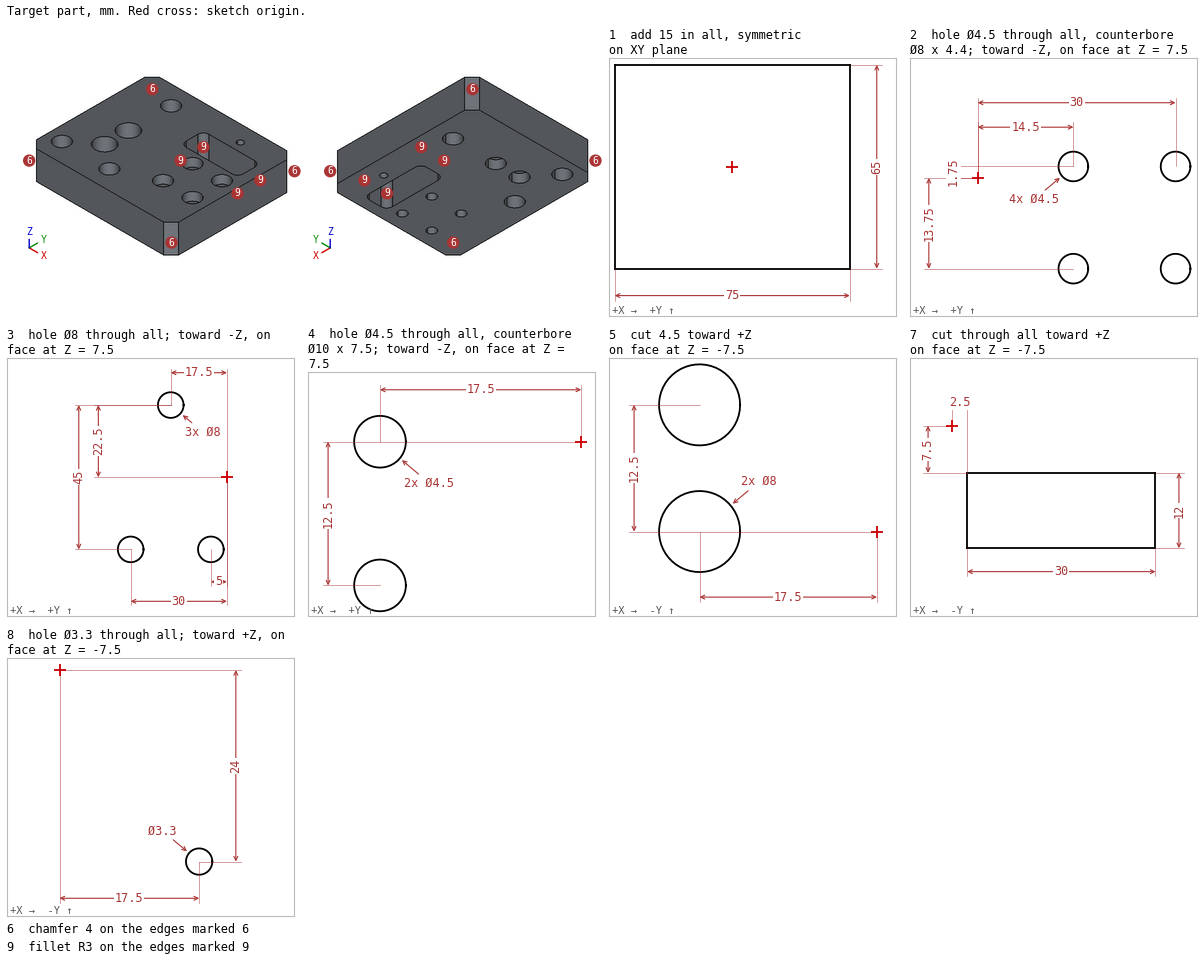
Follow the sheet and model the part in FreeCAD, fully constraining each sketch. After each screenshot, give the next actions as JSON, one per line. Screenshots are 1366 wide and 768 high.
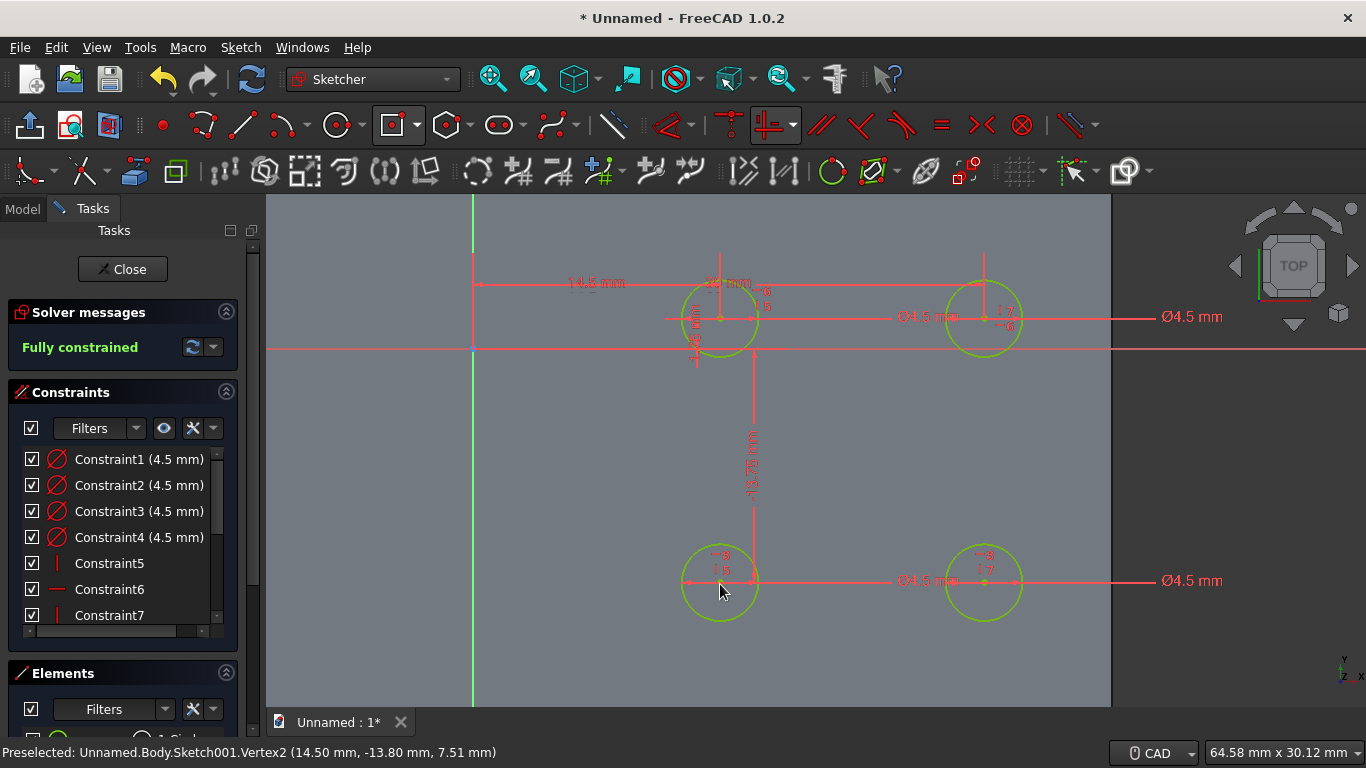
{"action": "left_click", "coordinate": [123, 269]}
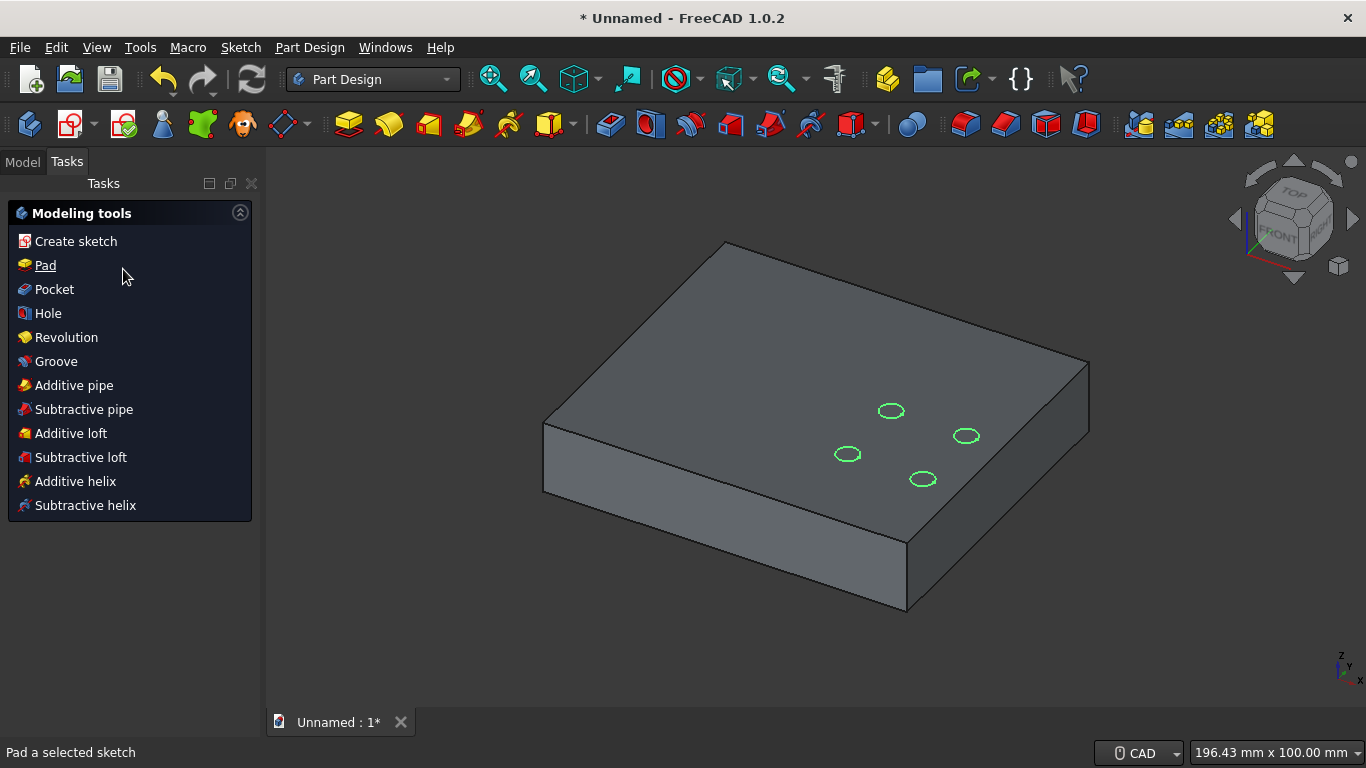
{"action": "left_click", "coordinate": [652, 124]}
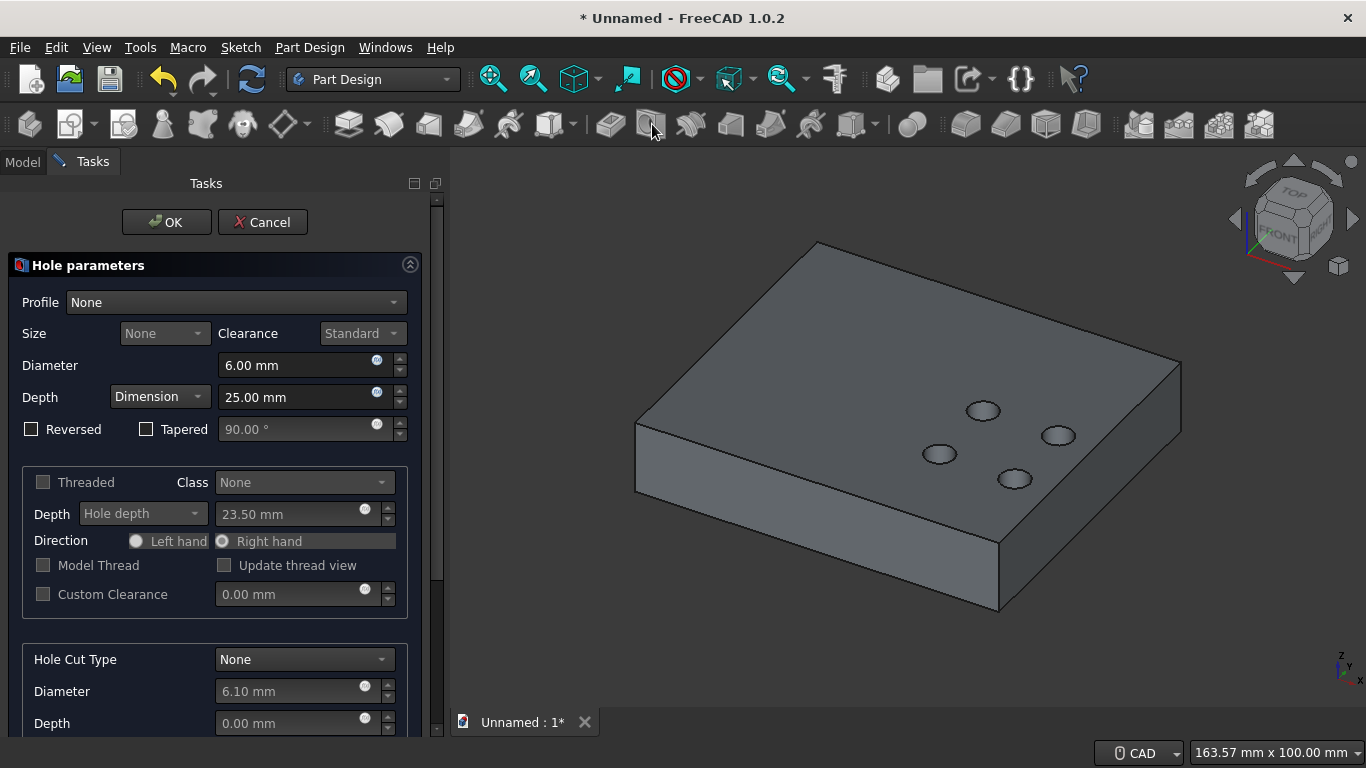
{"action": "triple_click", "coordinate": [305, 365]}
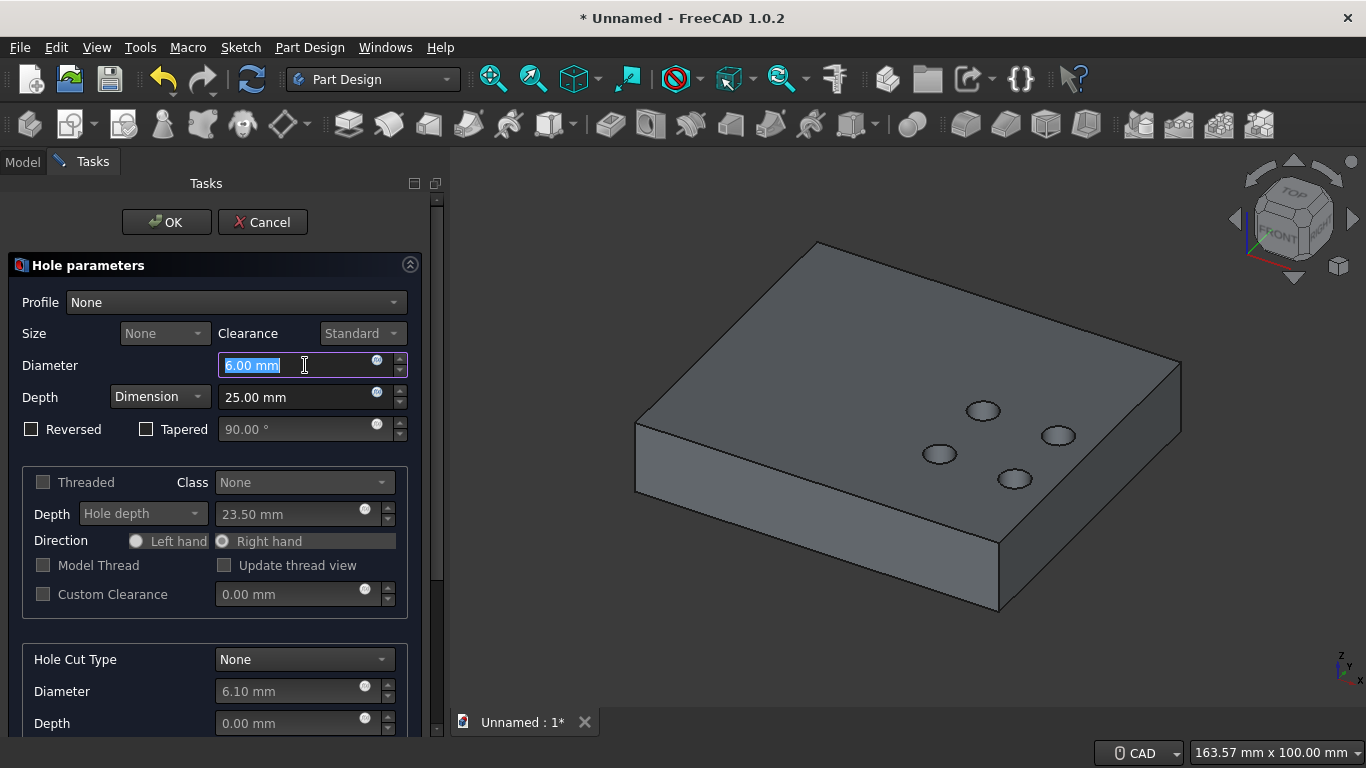
{"action": "type", "text": "4.5"}
{"action": "key", "text": "Tab"}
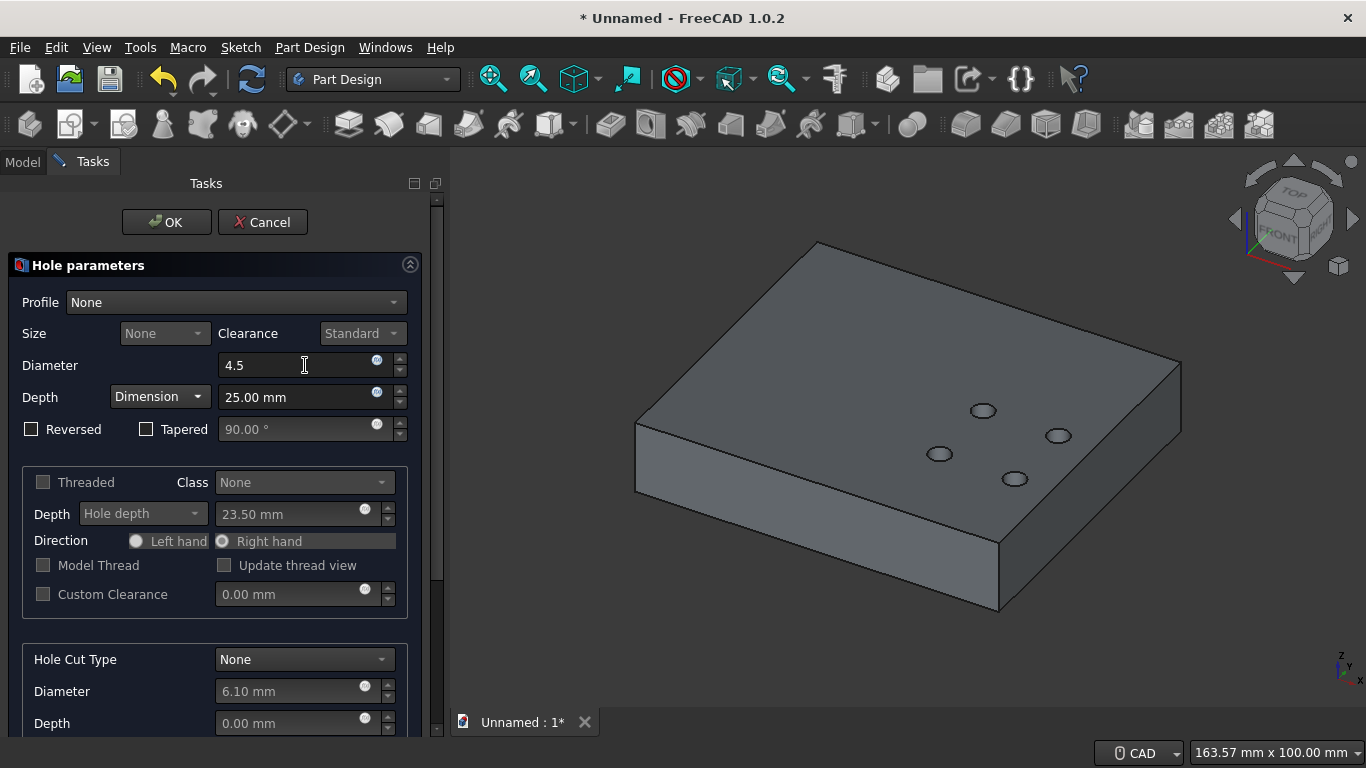
{"action": "left_click", "coordinate": [161, 396]}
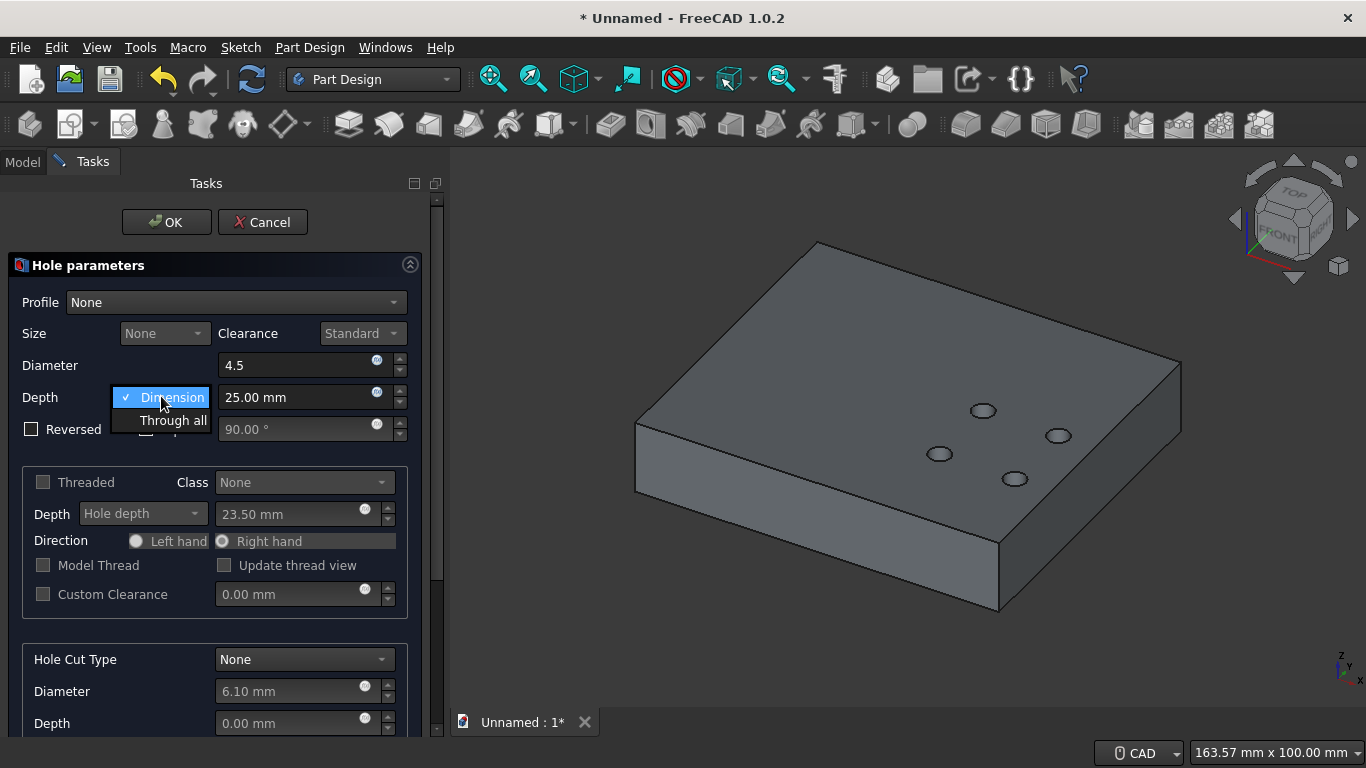
{"action": "left_click", "coordinate": [160, 420]}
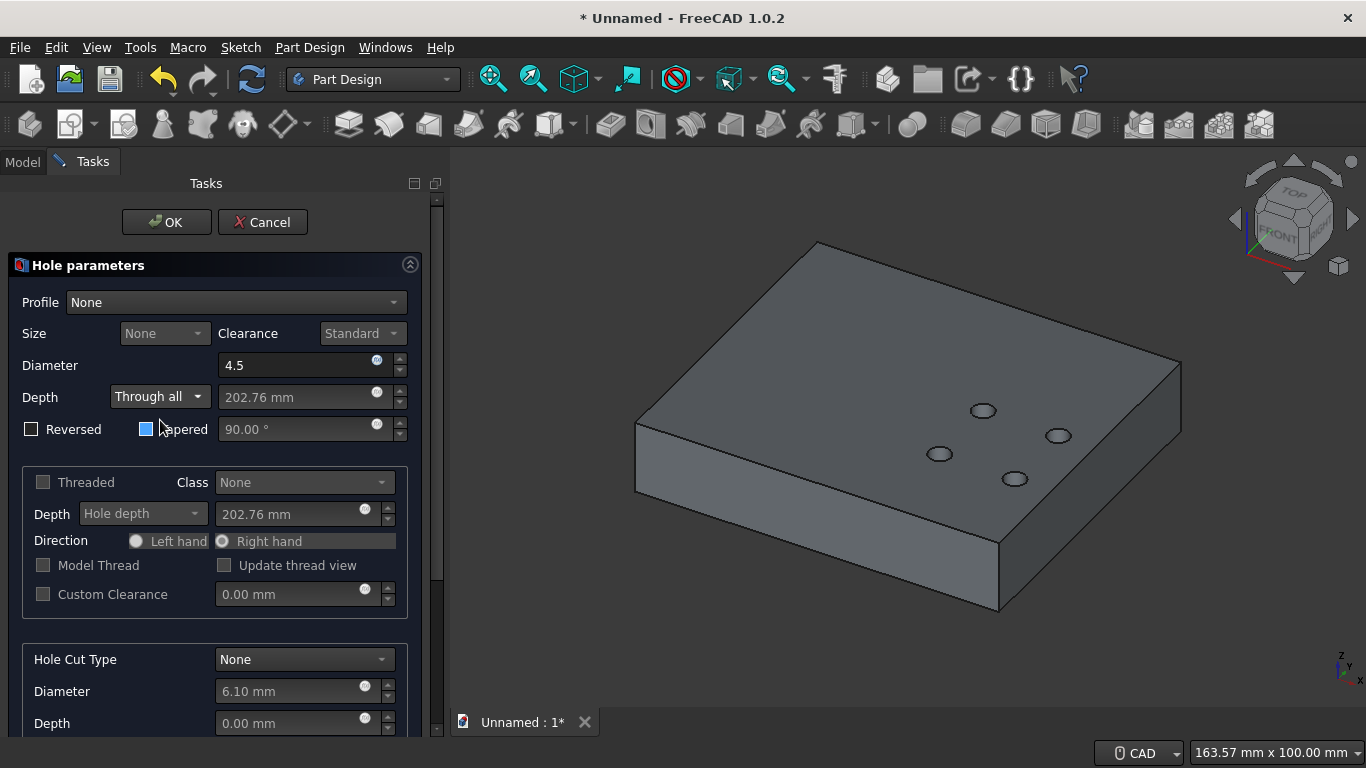
{"action": "left_click", "coordinate": [306, 660]}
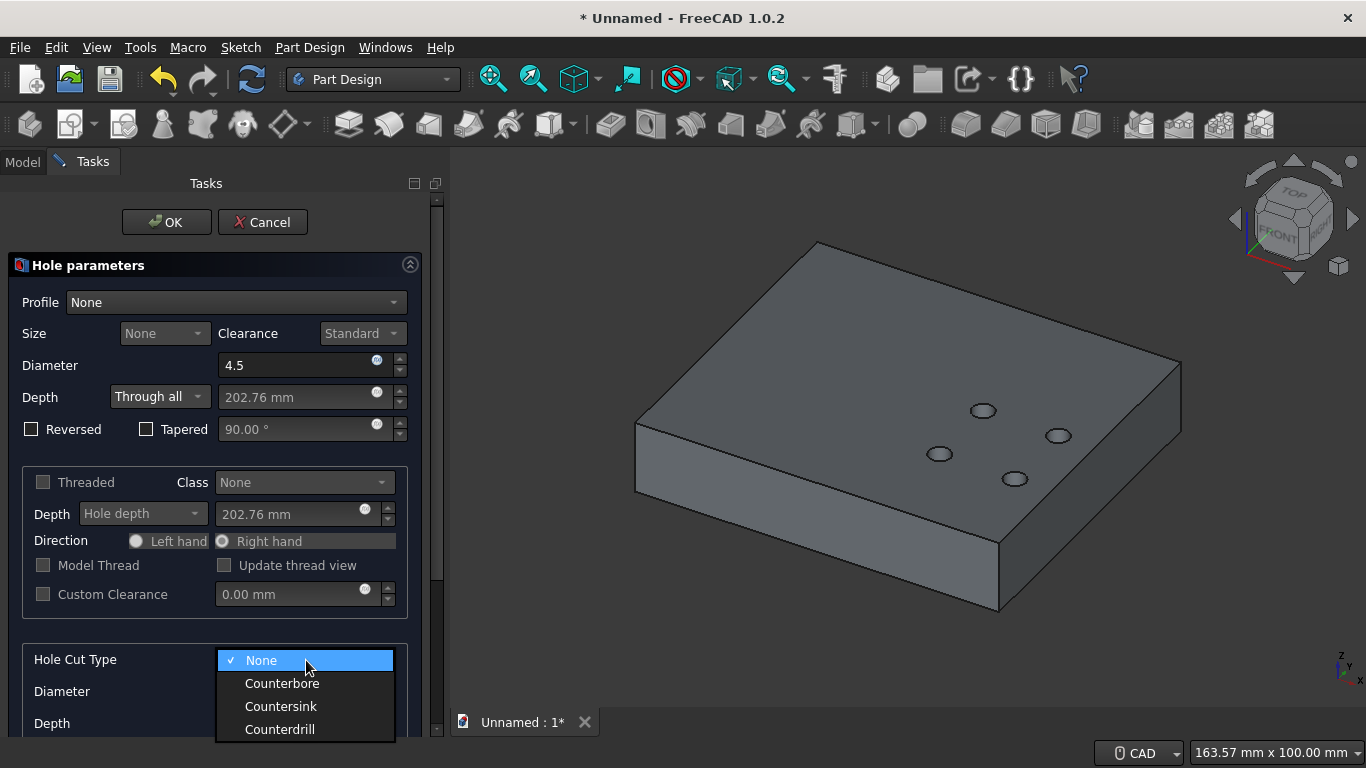
{"action": "left_click", "coordinate": [304, 684]}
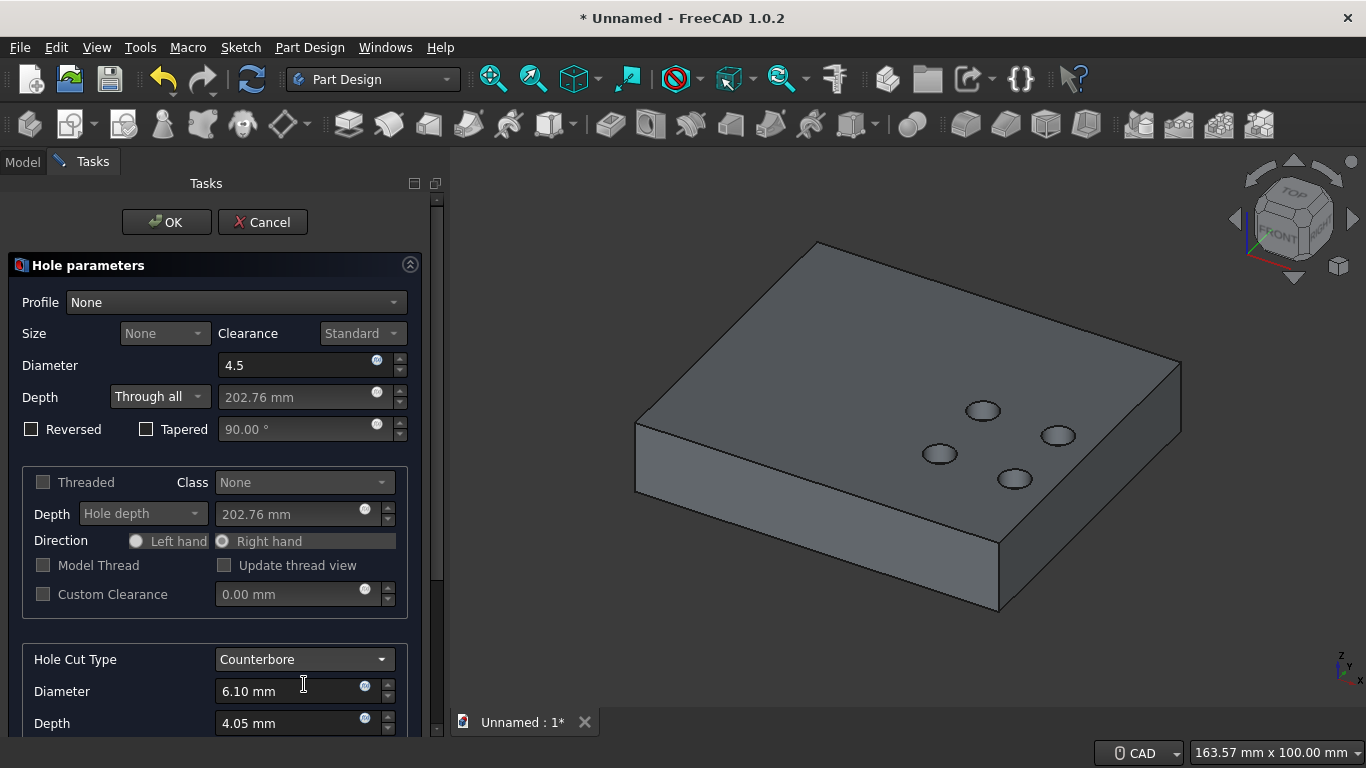
{"action": "triple_click", "coordinate": [298, 691]}